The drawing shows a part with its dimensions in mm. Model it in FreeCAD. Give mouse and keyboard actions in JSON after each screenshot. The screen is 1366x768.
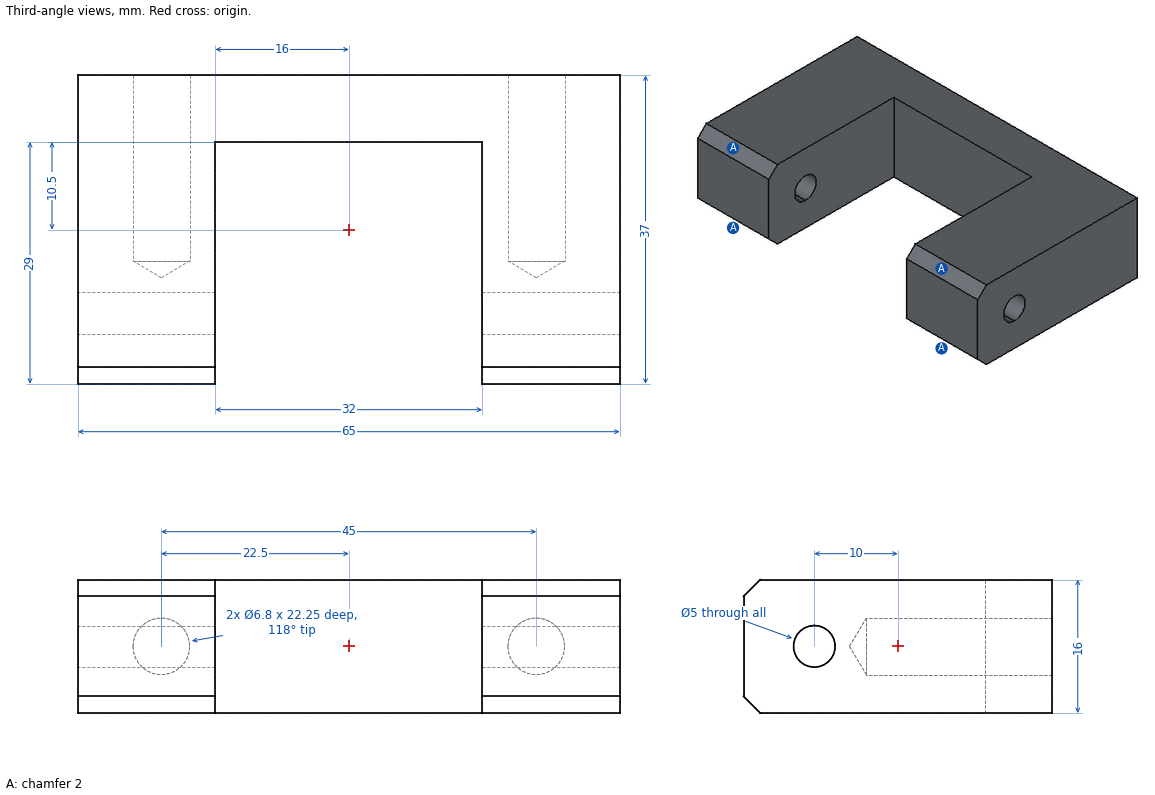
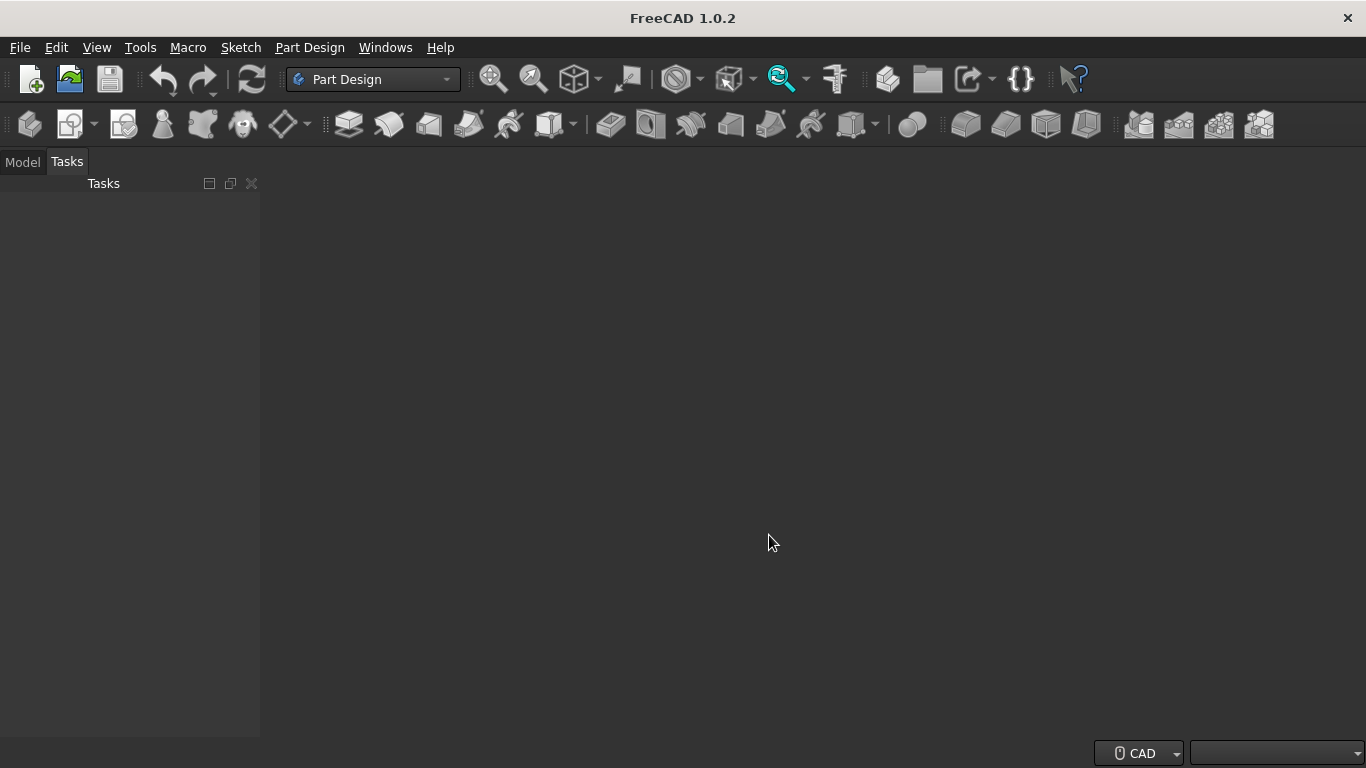
{"action": "left_click", "coordinate": [30, 80]}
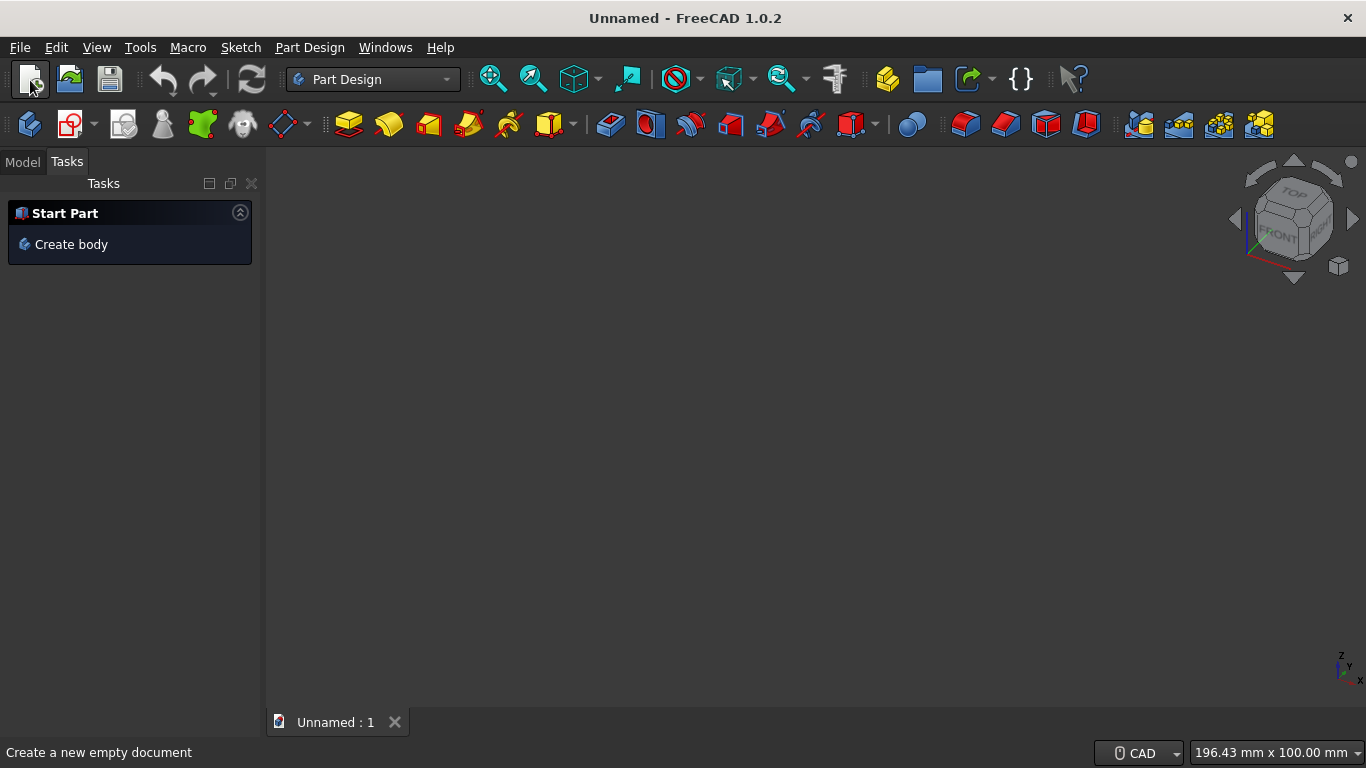
{"action": "left_click", "coordinate": [70, 124]}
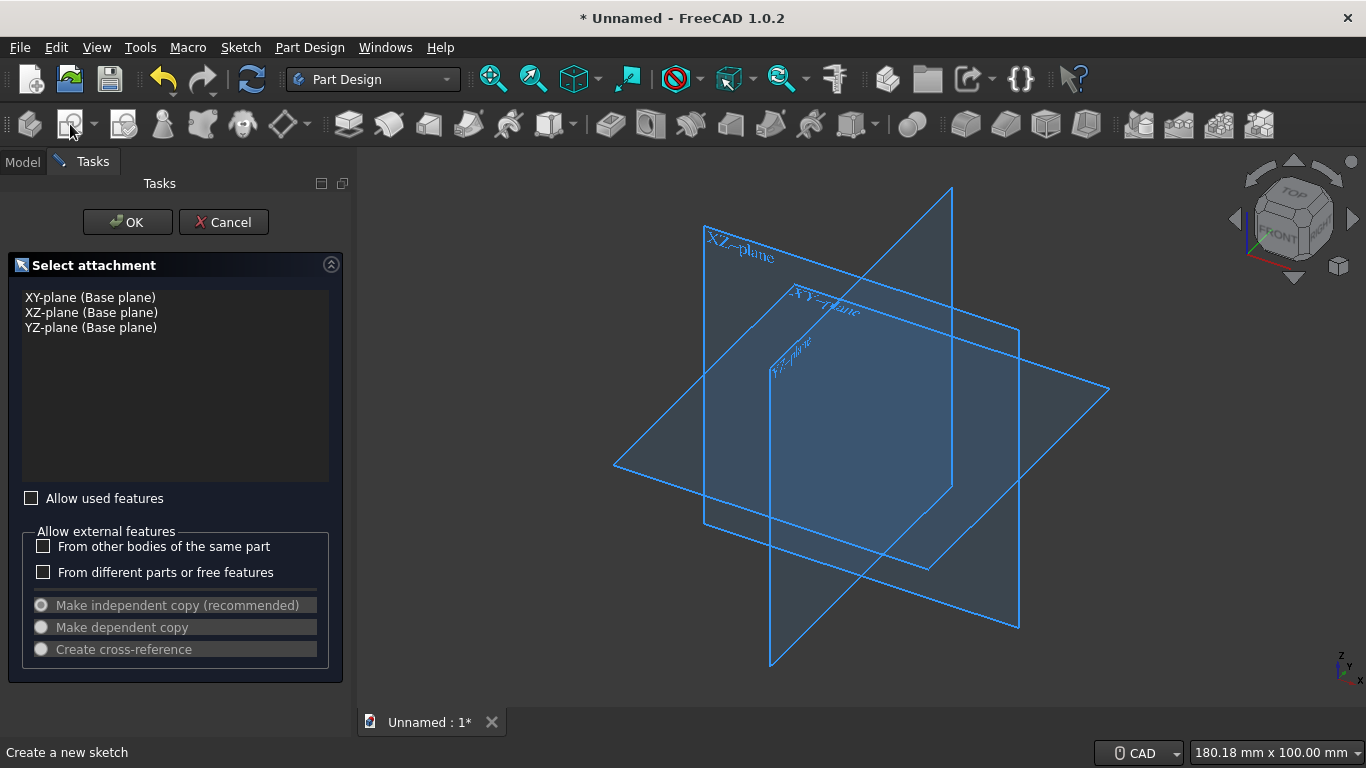
{"action": "left_click", "coordinate": [82, 298]}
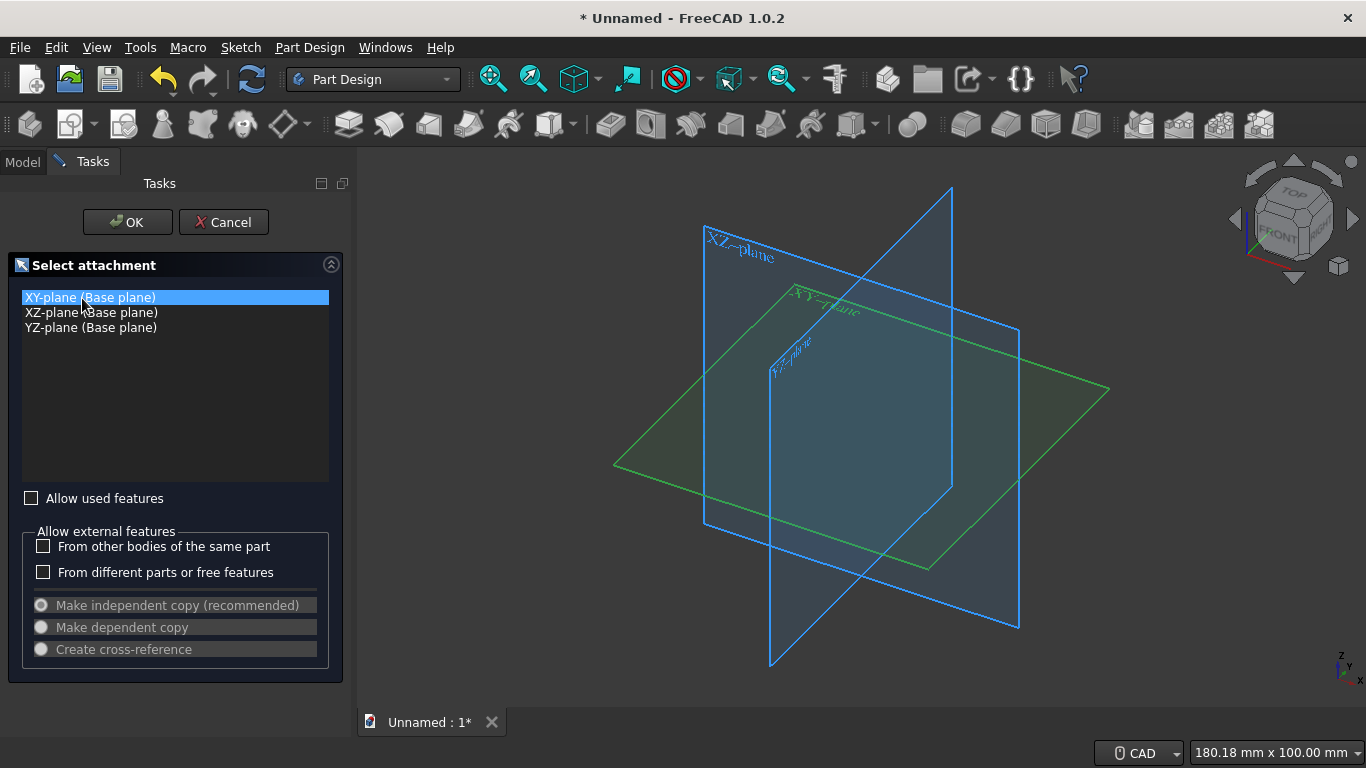
{"action": "left_click", "coordinate": [128, 222]}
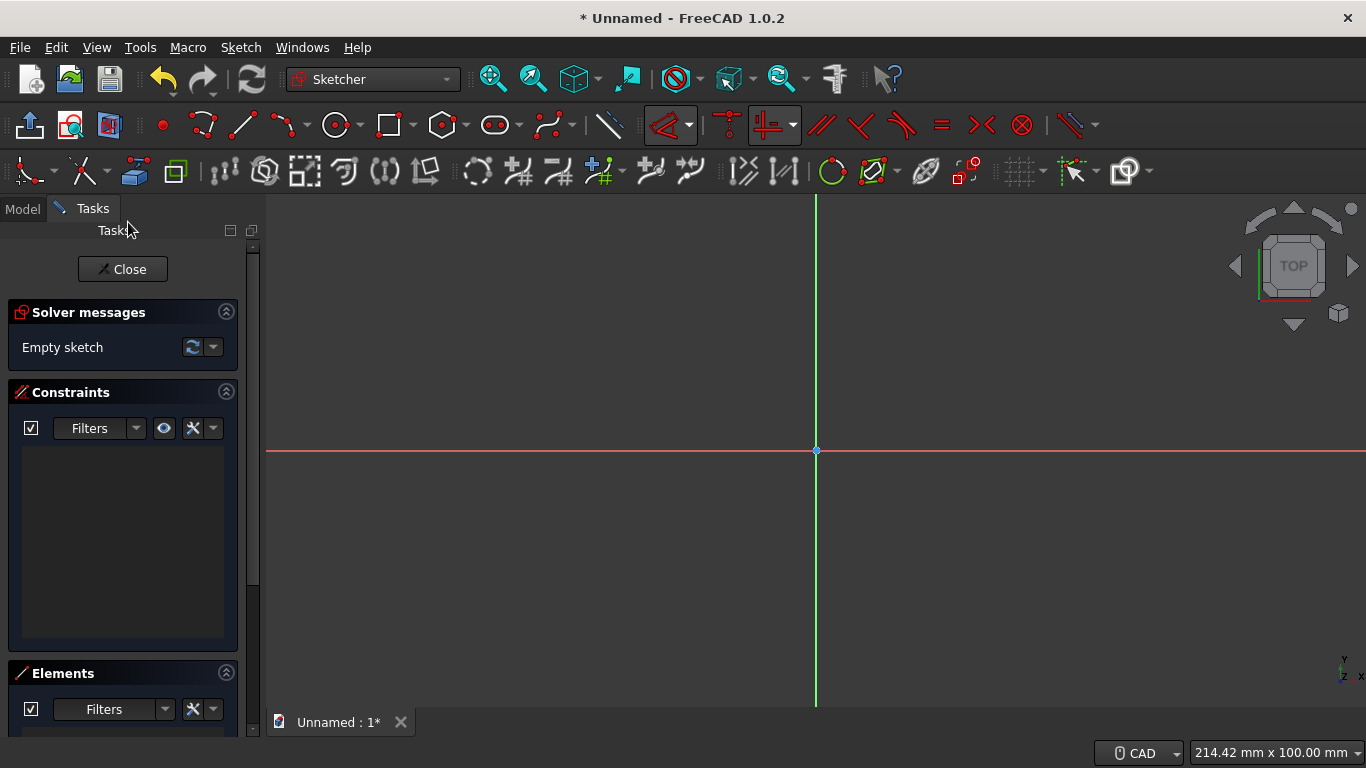
{"action": "scroll", "coordinate": [899, 450], "scroll_direction": "up", "scroll_amount": 3}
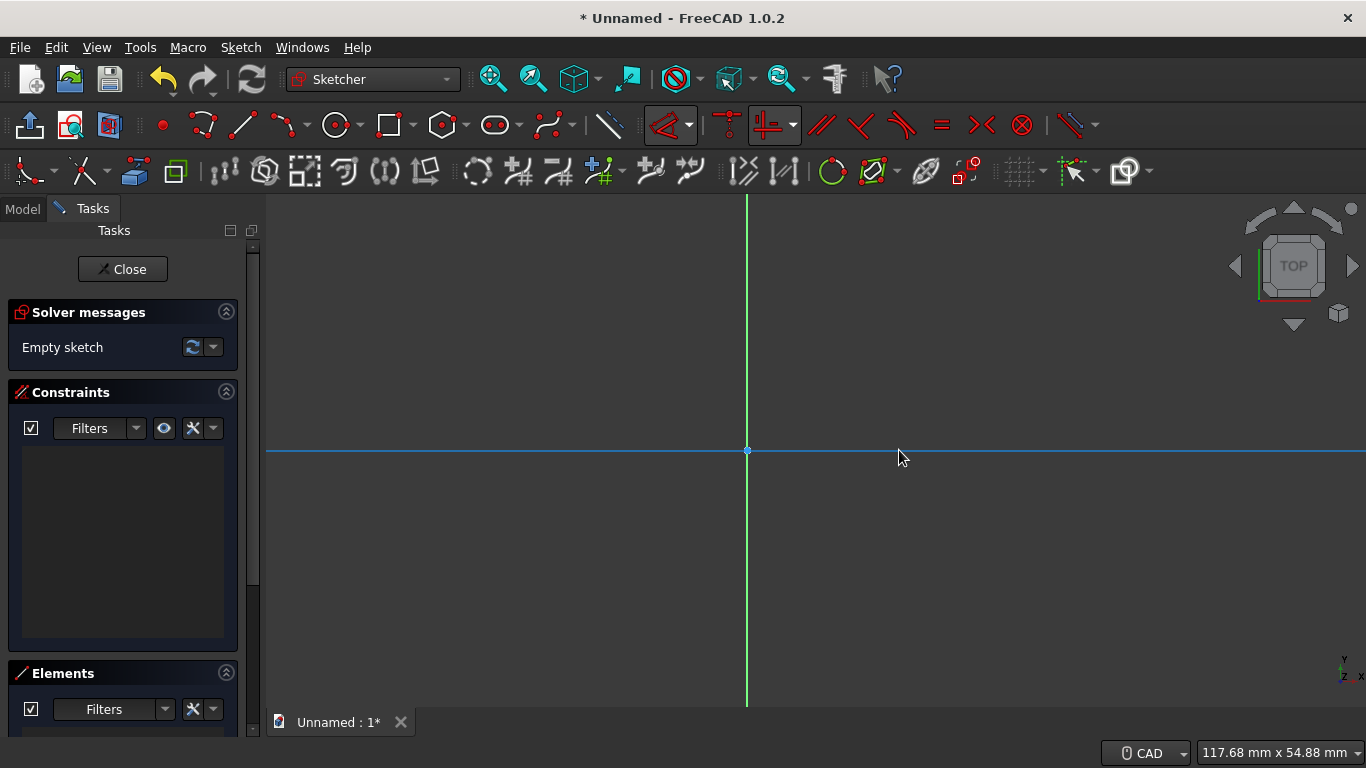
{"action": "left_click", "coordinate": [416, 126]}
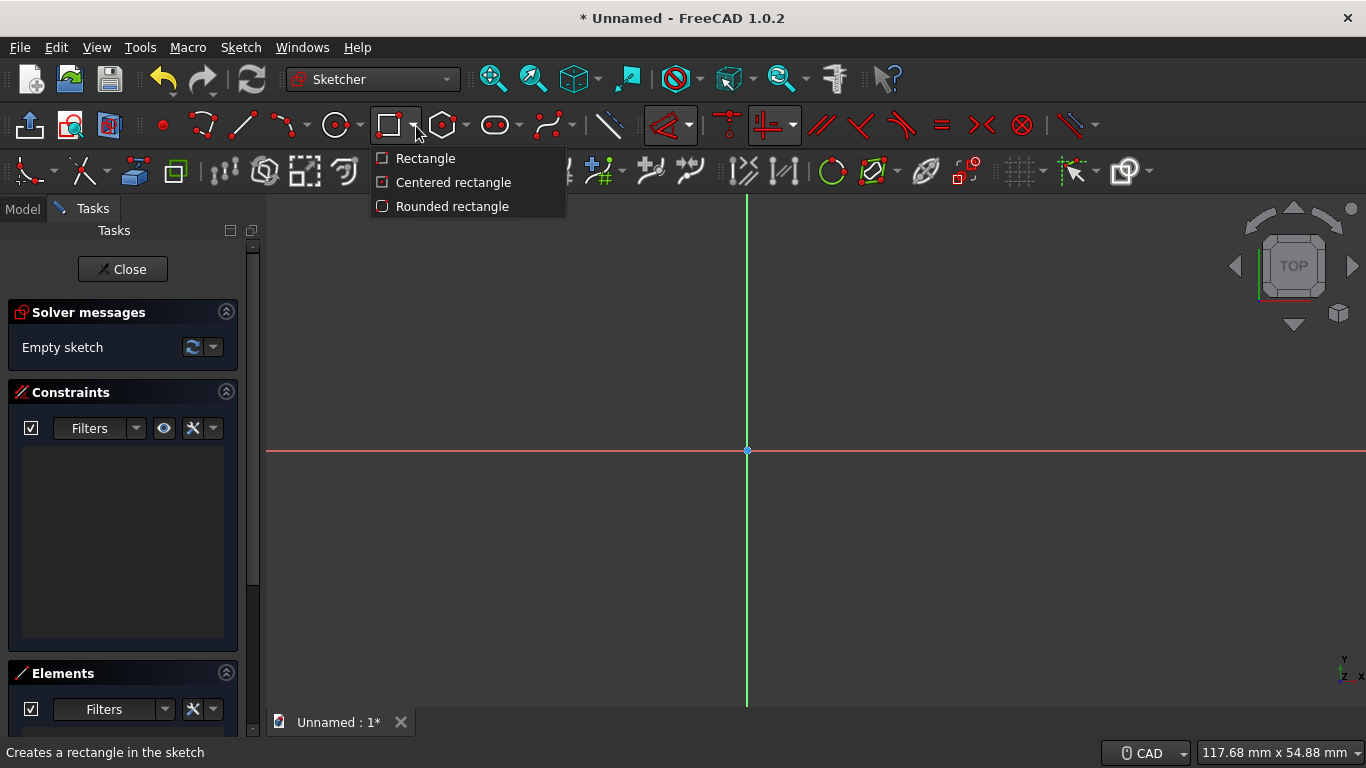
{"action": "left_click", "coordinate": [468, 182]}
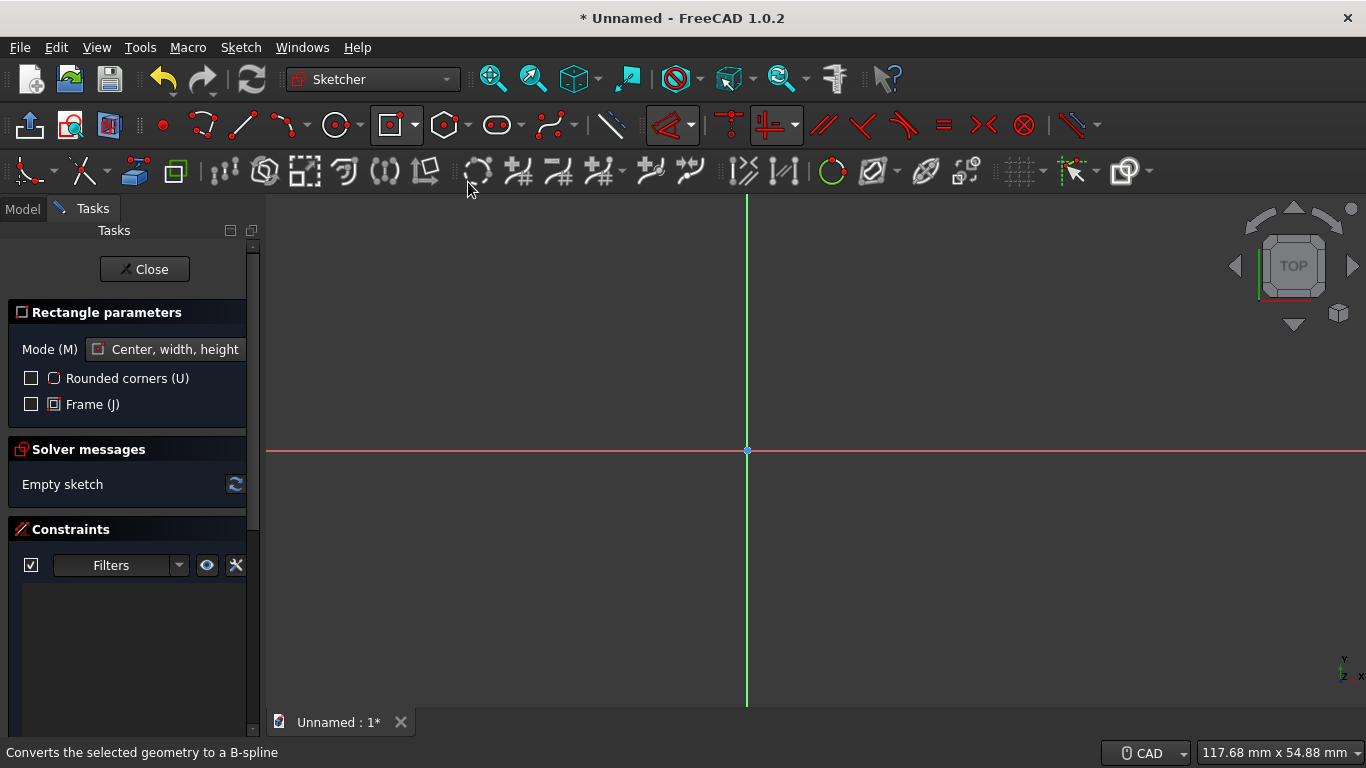
{"action": "left_click", "coordinate": [747, 450]}
{"action": "left_click", "coordinate": [1051, 278]}
{"action": "key", "text": "Escape"}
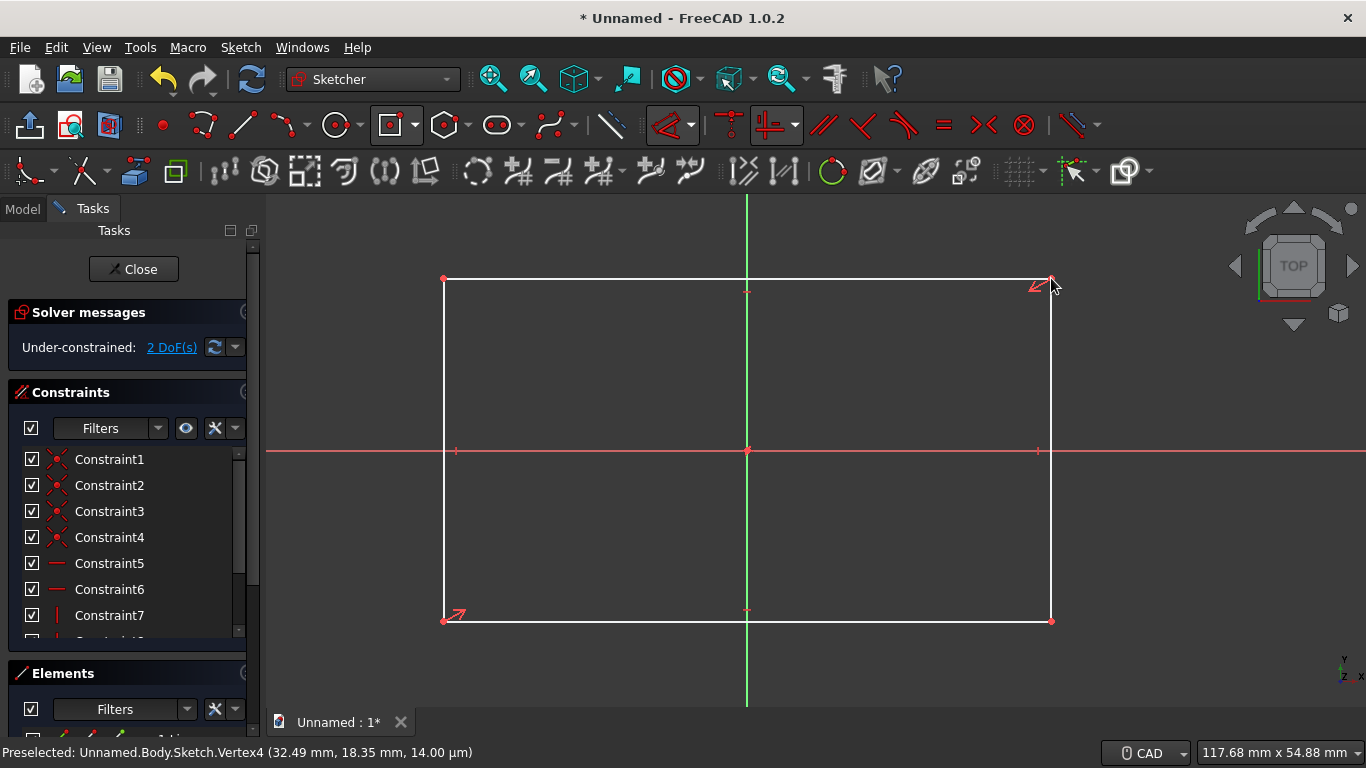
{"action": "left_click", "coordinate": [626, 622]}